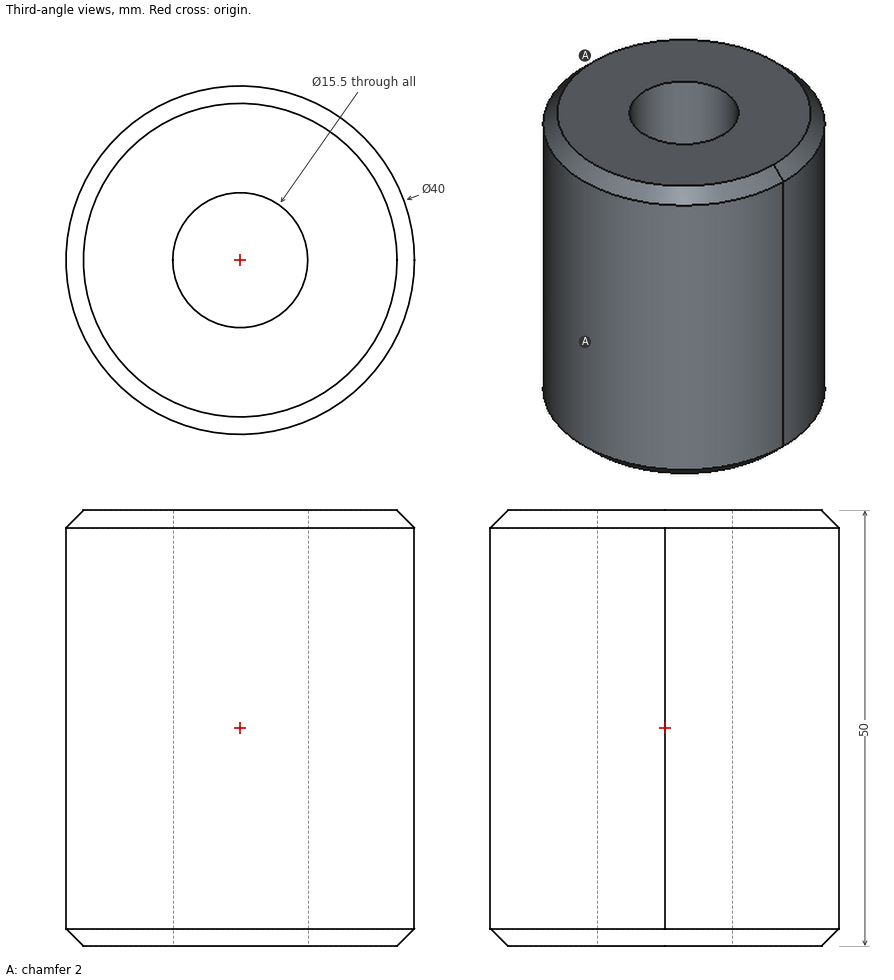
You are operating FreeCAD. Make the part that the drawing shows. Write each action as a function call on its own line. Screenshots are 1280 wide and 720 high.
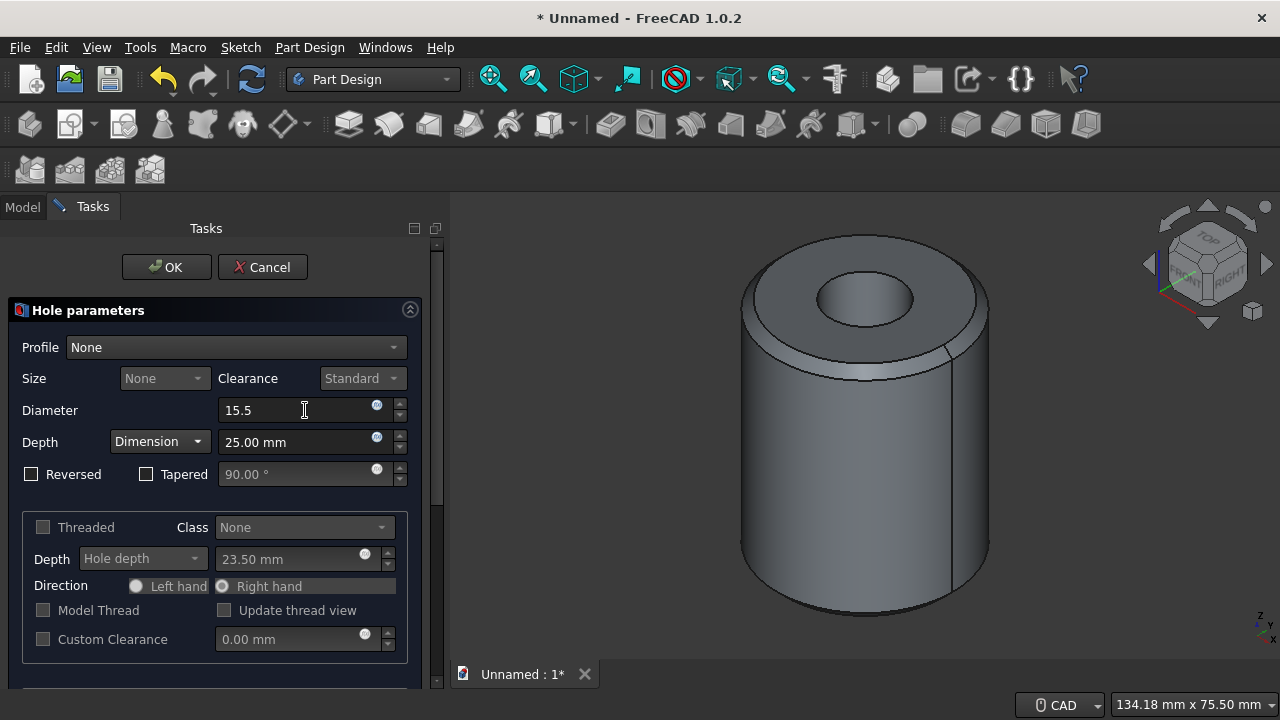
click(161, 442)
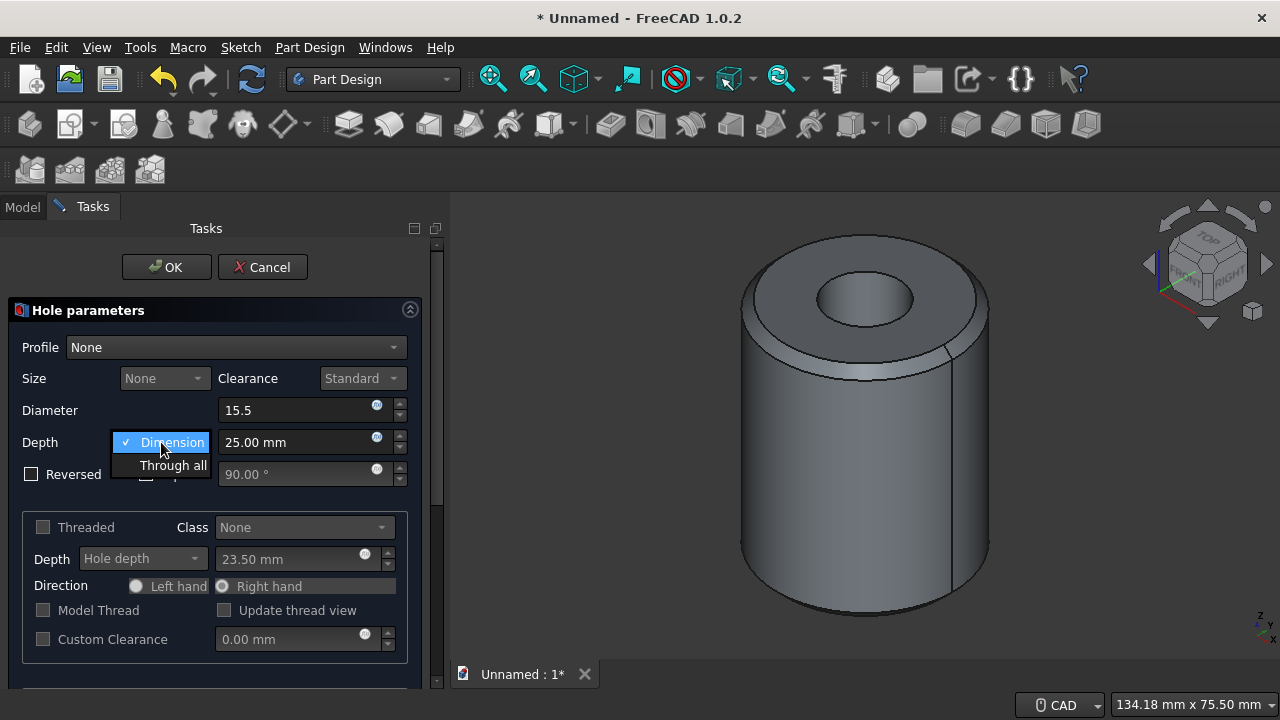
click(160, 466)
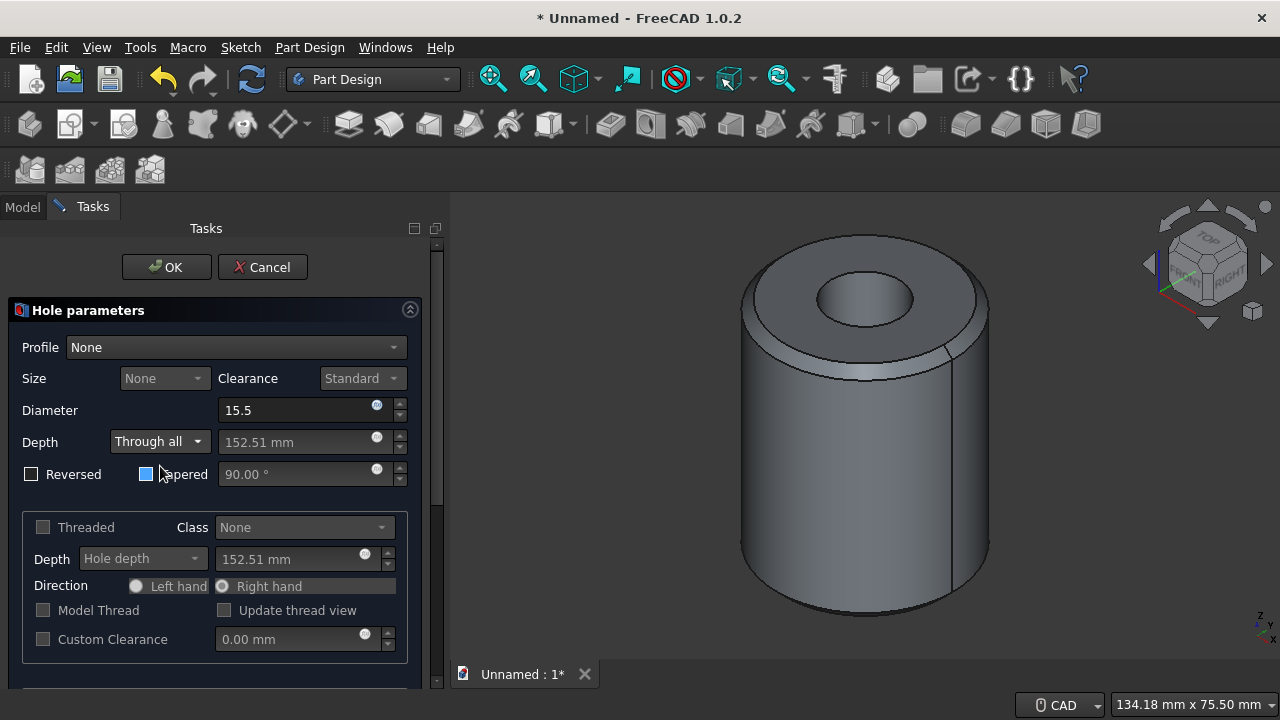
click(167, 267)